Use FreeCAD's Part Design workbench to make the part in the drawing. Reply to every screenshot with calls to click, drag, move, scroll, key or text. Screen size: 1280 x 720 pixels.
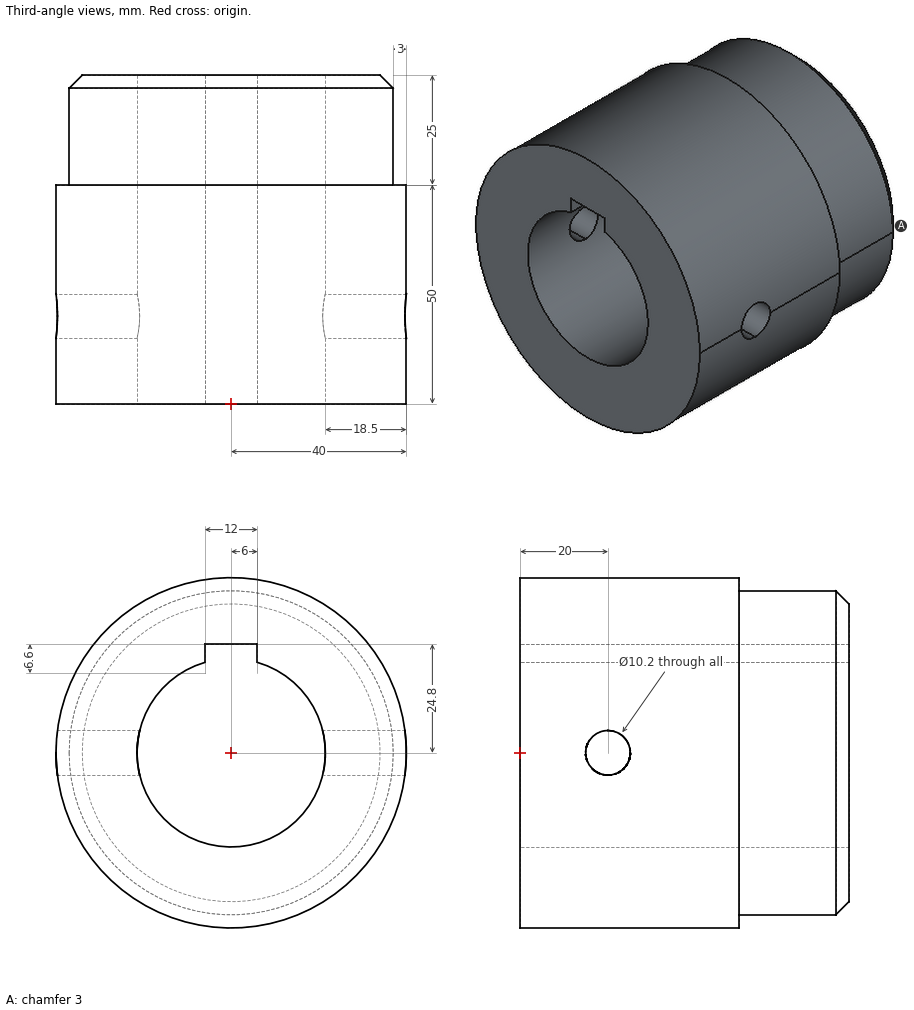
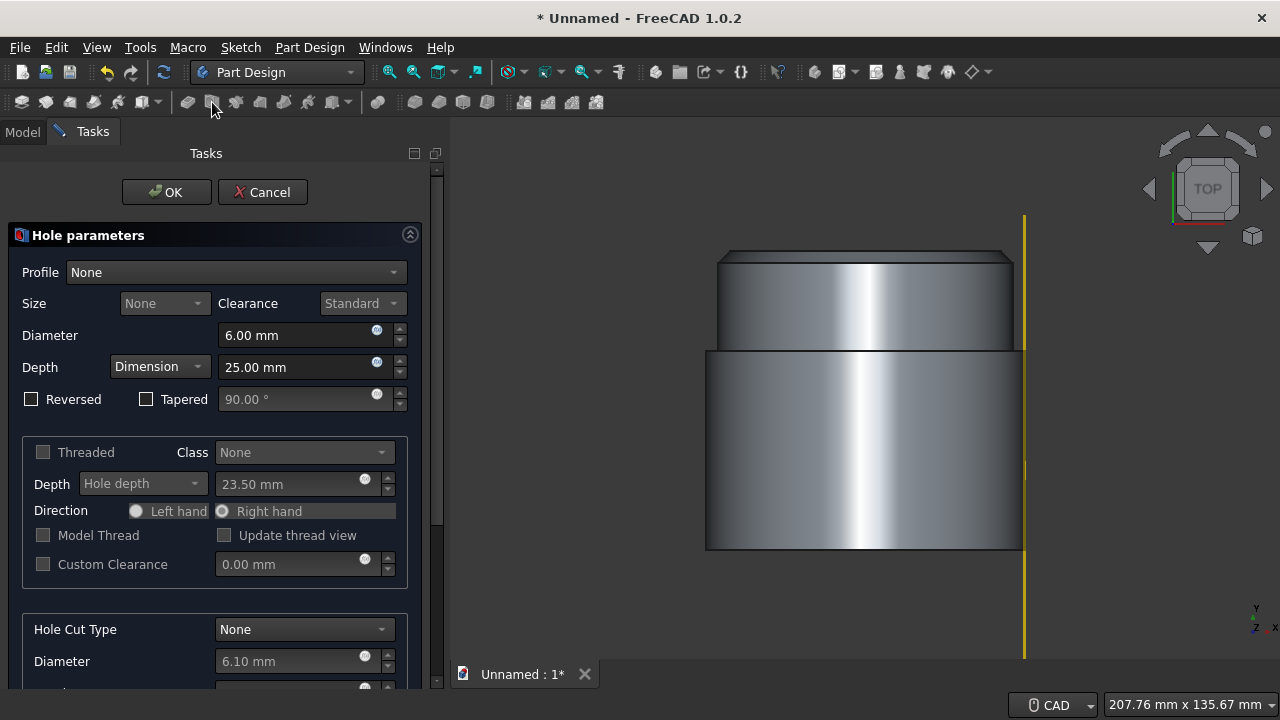
triple_click(305, 335)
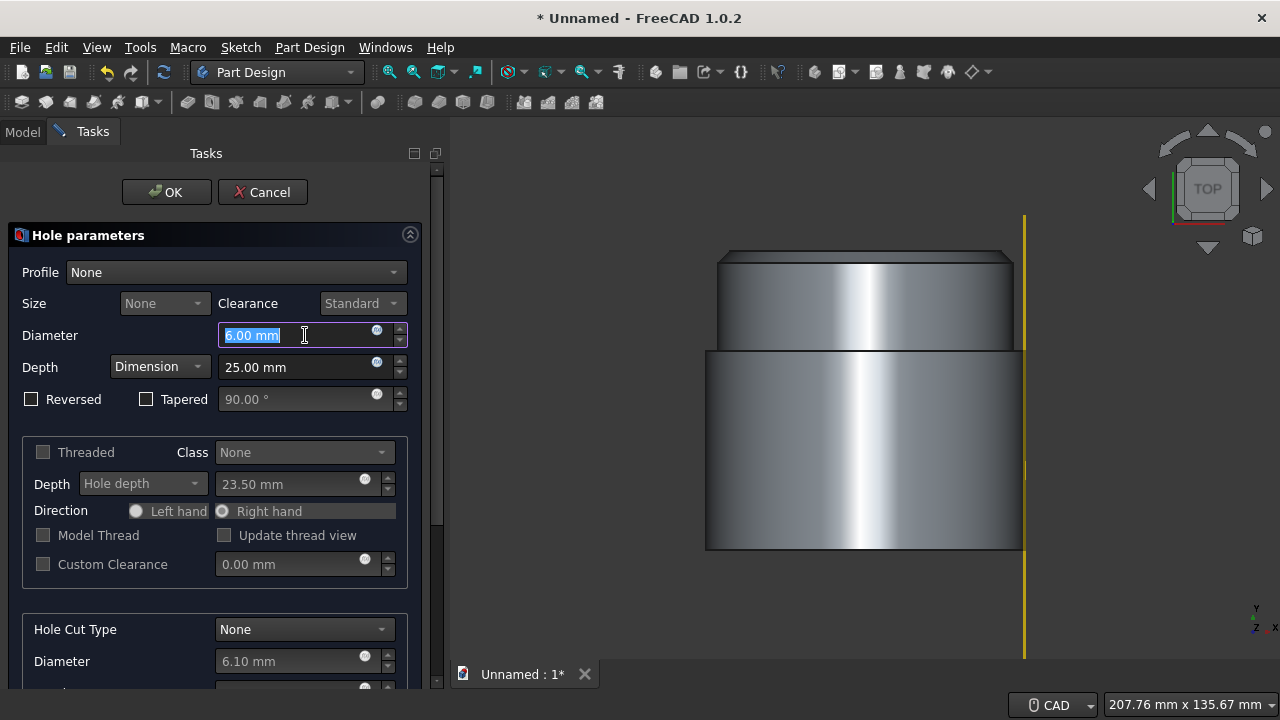
text(10.2)
key(Tab)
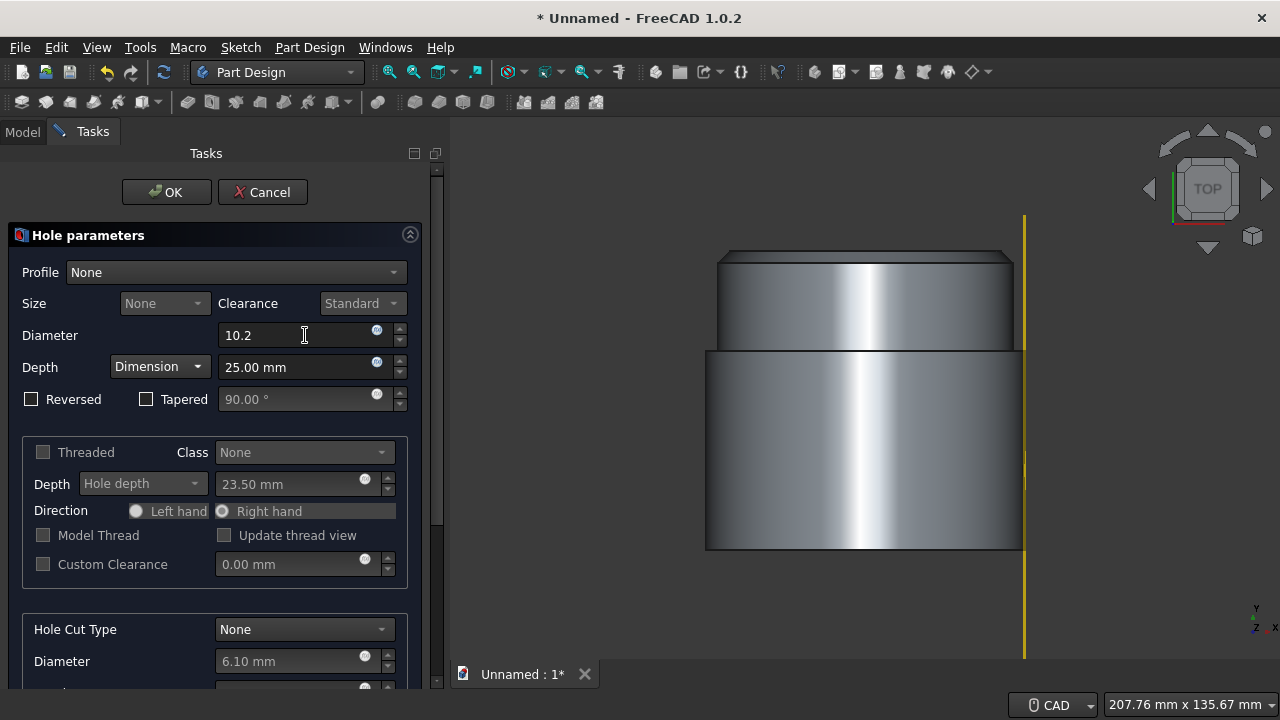
click(161, 366)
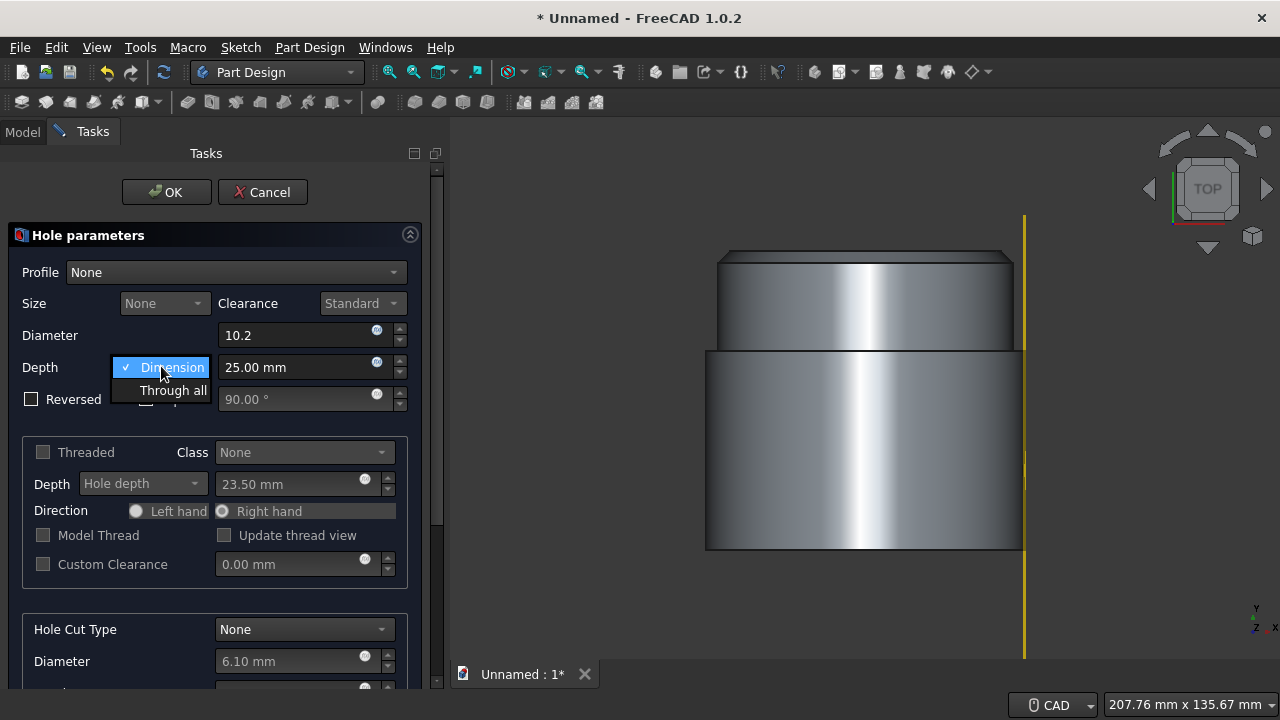
click(160, 390)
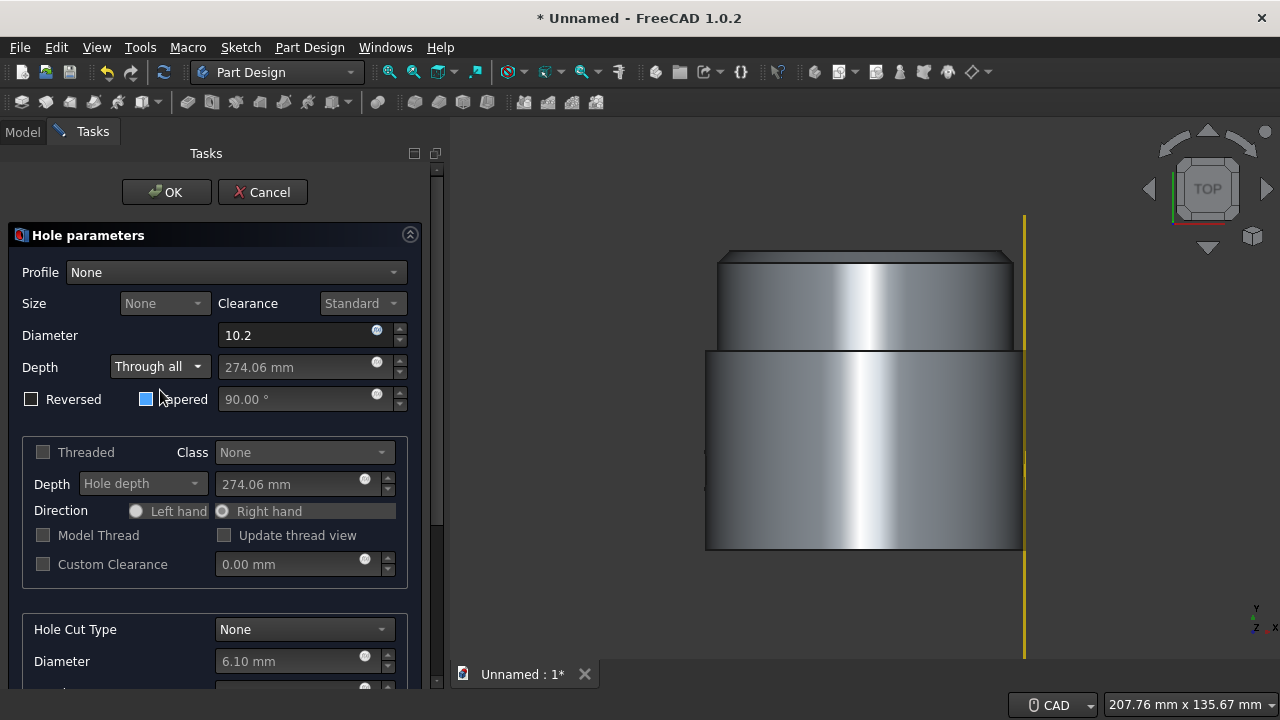
click(167, 192)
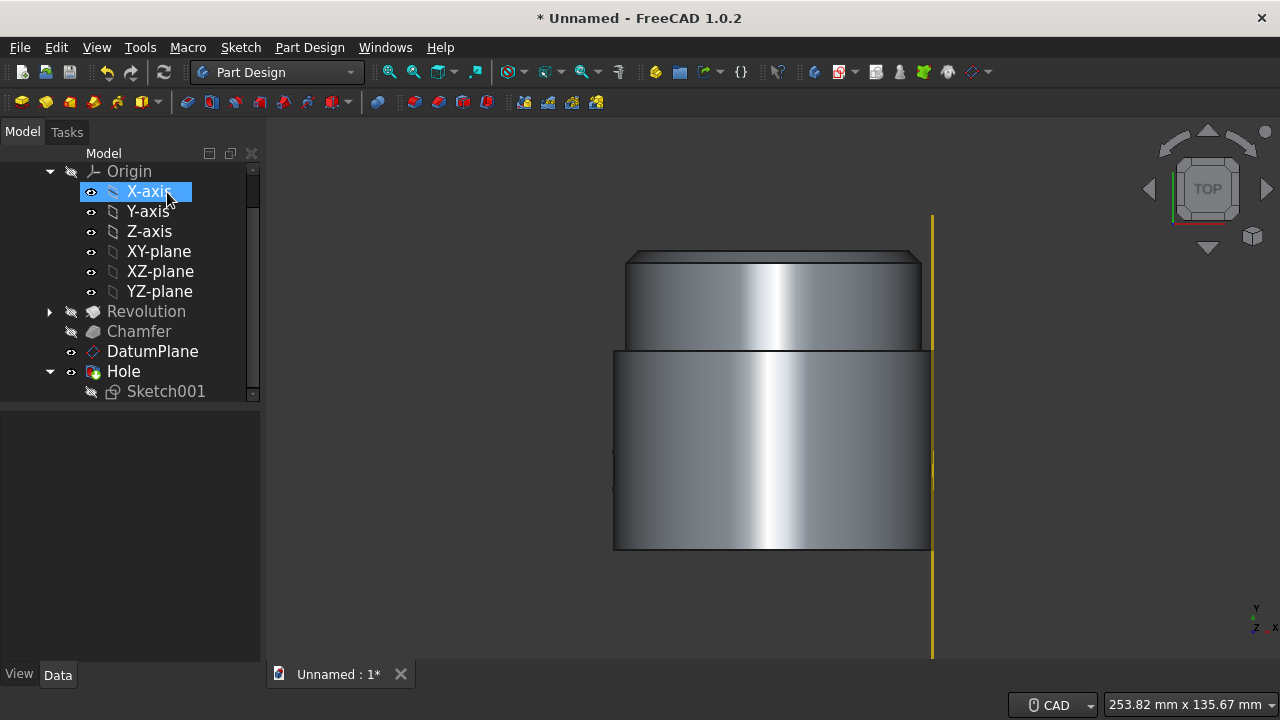
click(116, 352)
key(space)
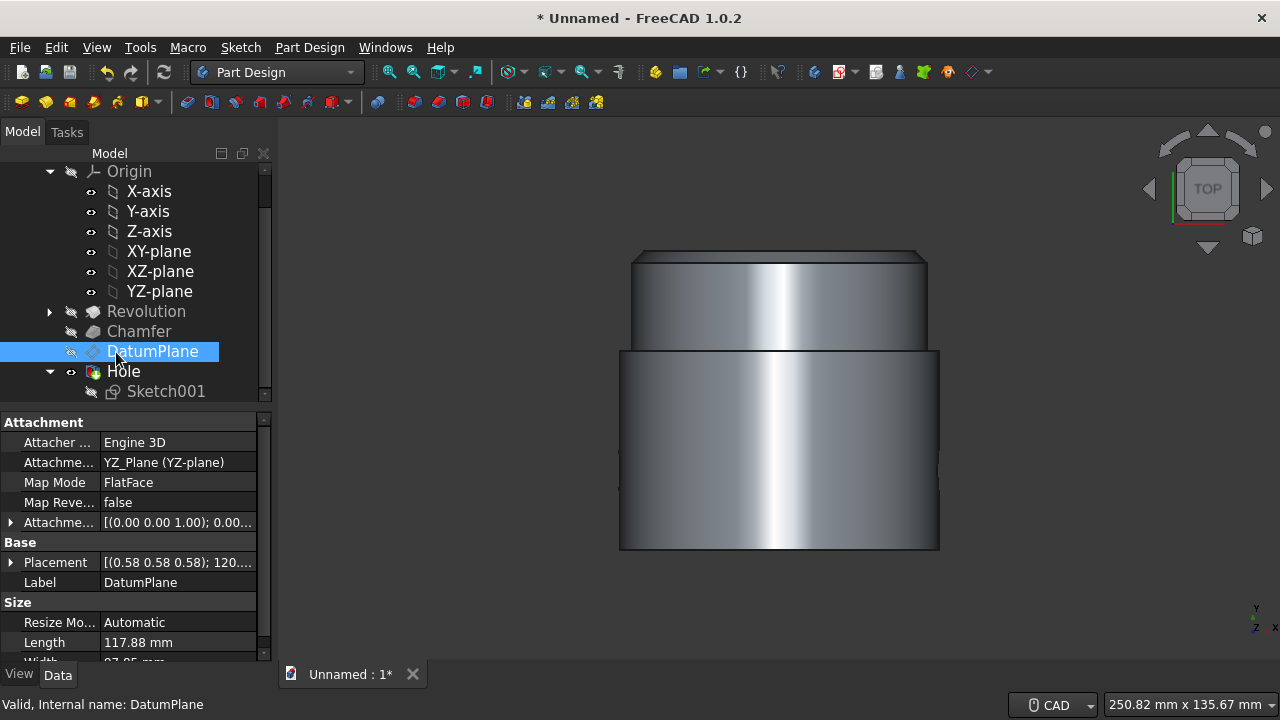
key(4)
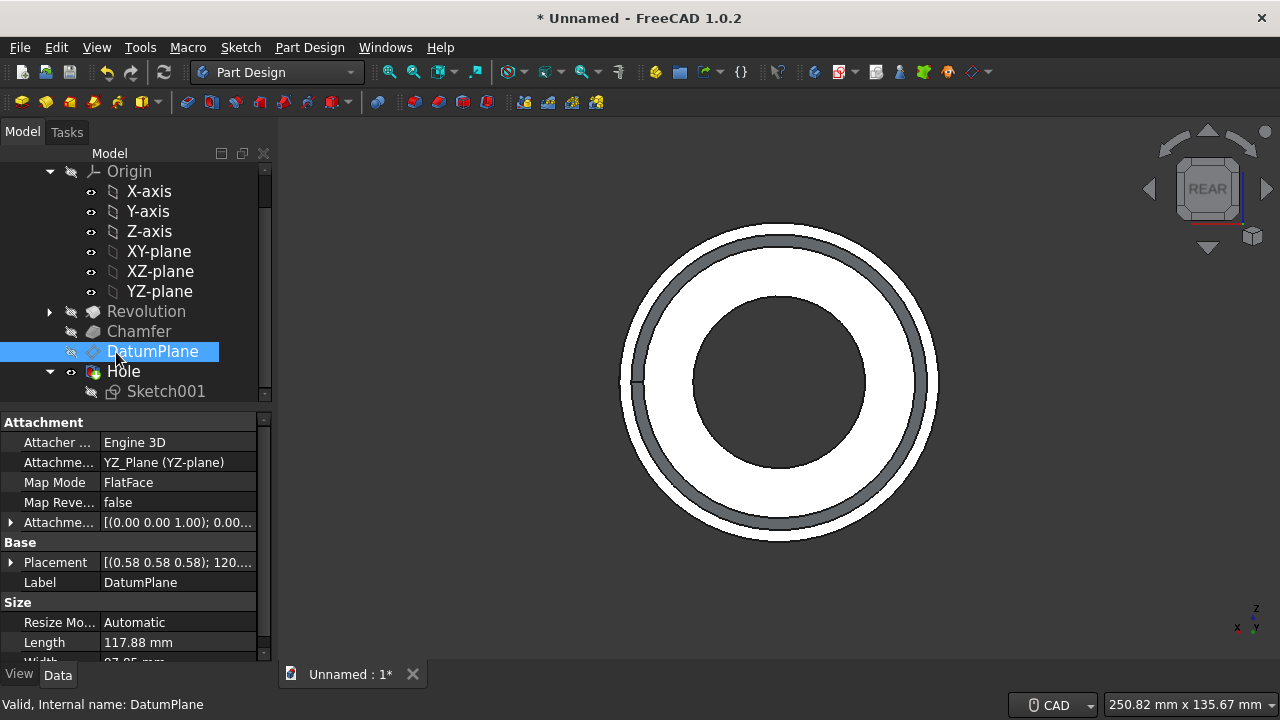
click(702, 304)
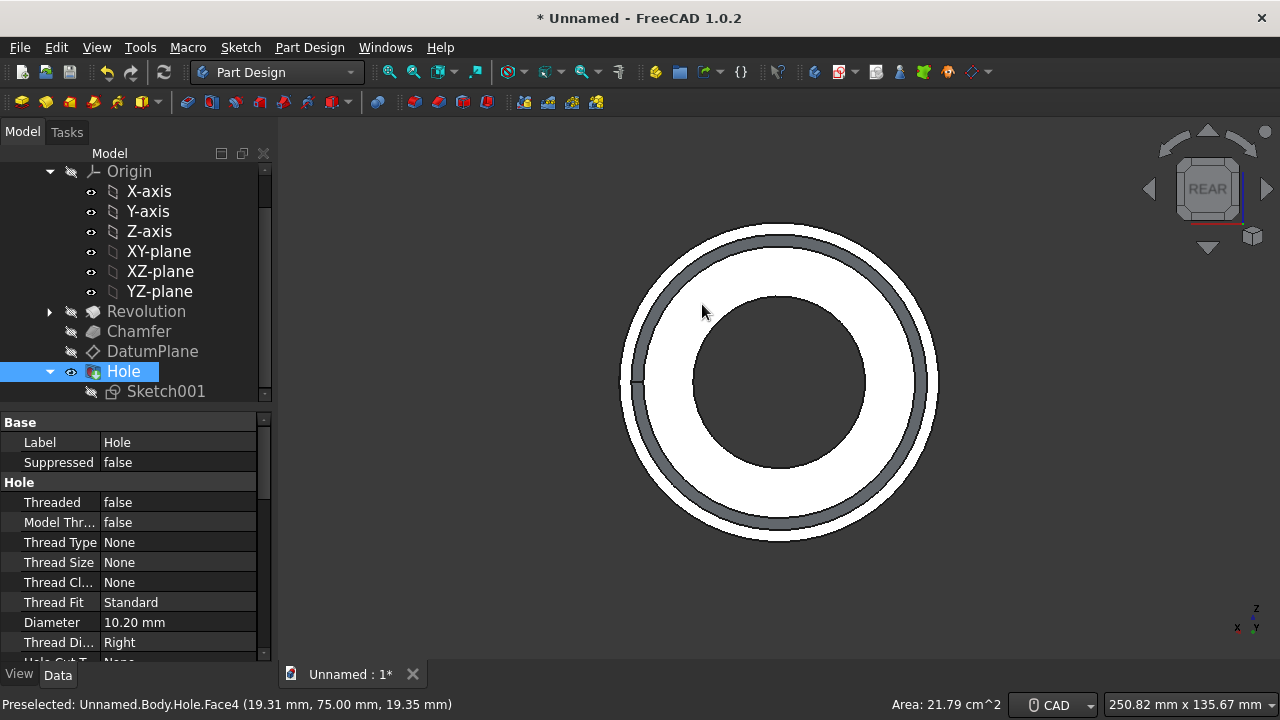
click(840, 72)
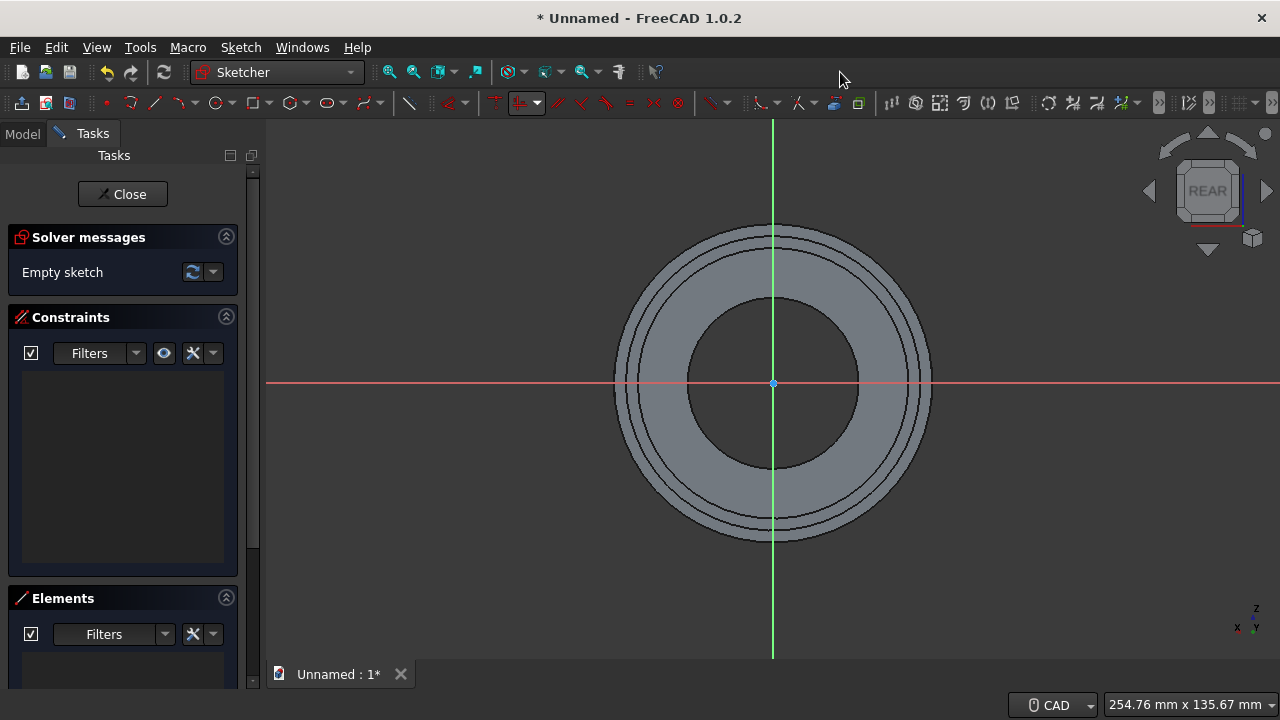
scroll(803, 310, up, 6)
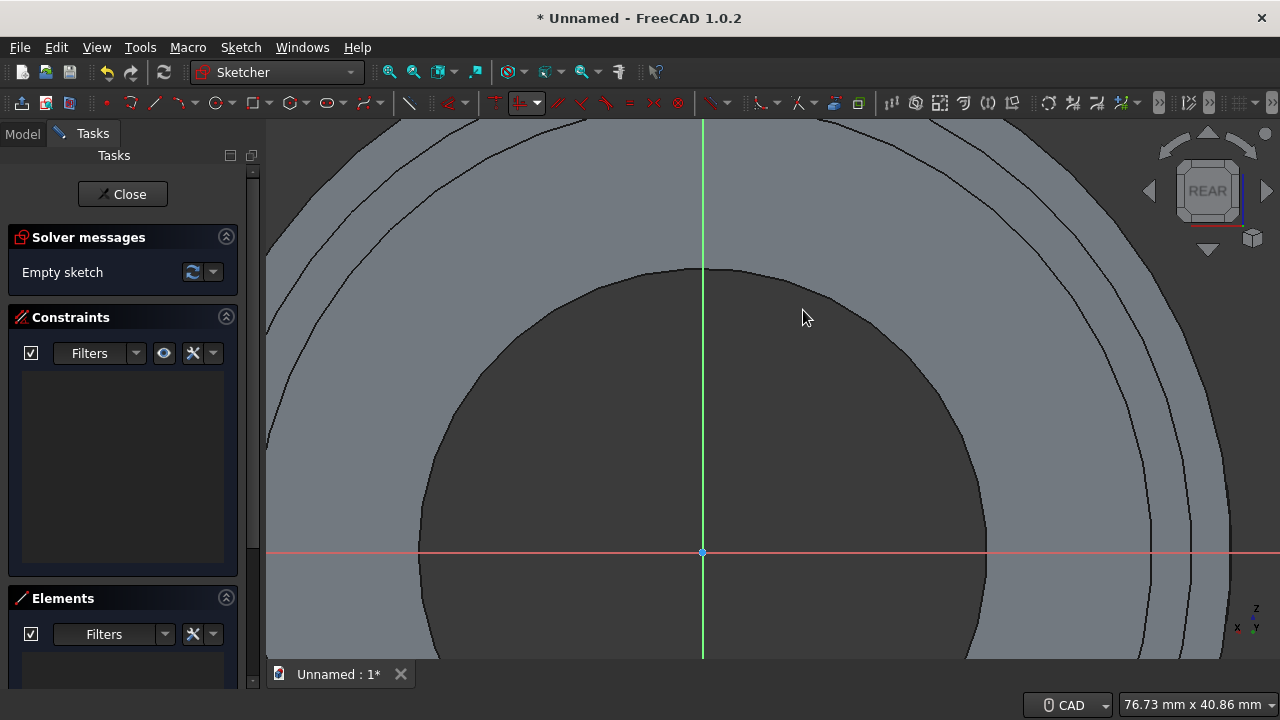
key(g)
key(r)